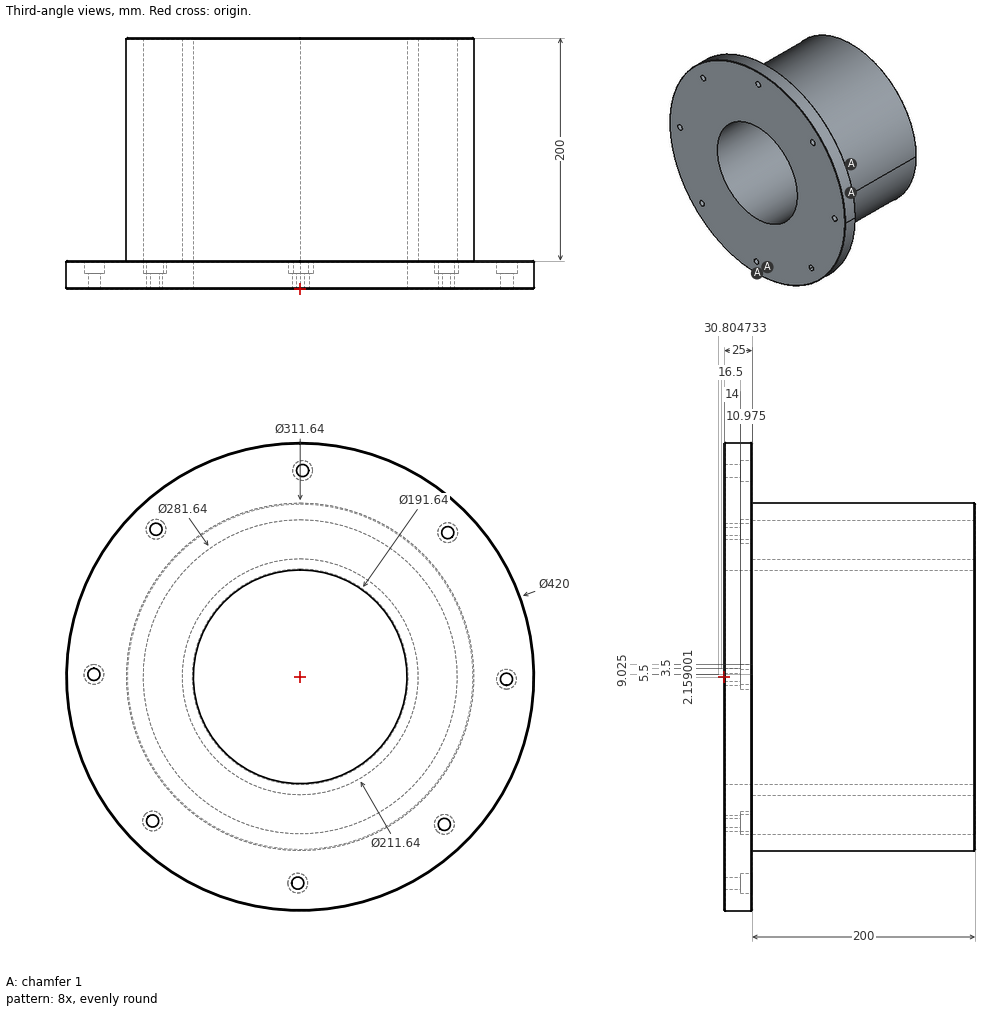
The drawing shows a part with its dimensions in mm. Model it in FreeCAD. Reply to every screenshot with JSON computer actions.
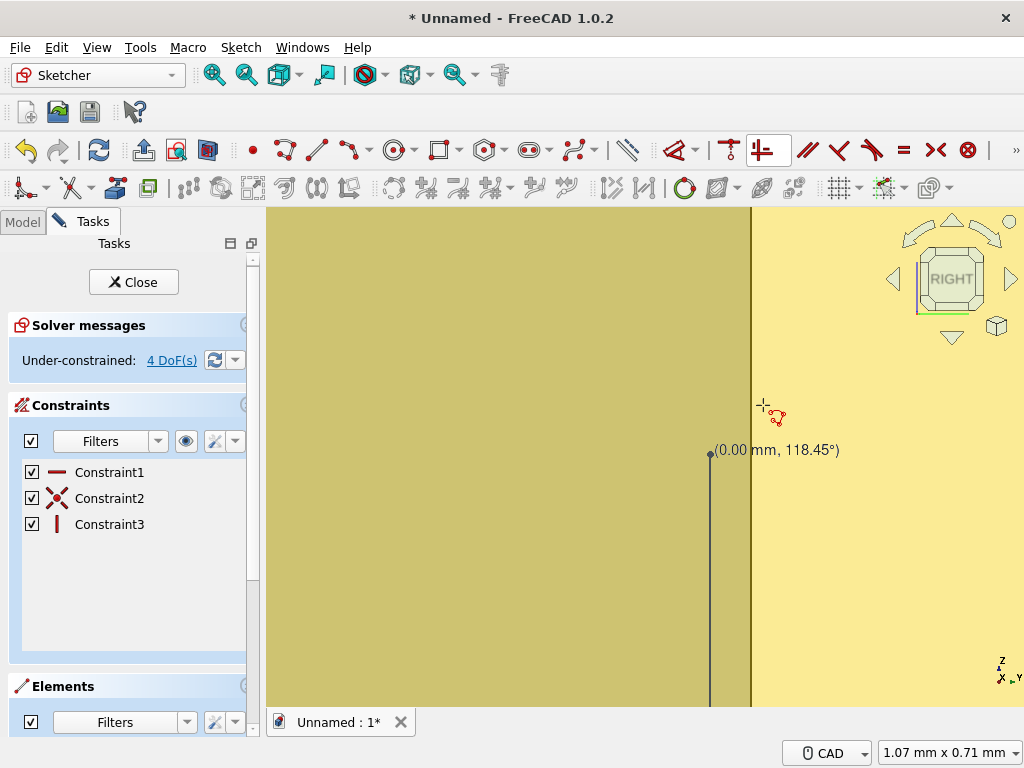
{"action": "left_click", "coordinate": [733, 398]}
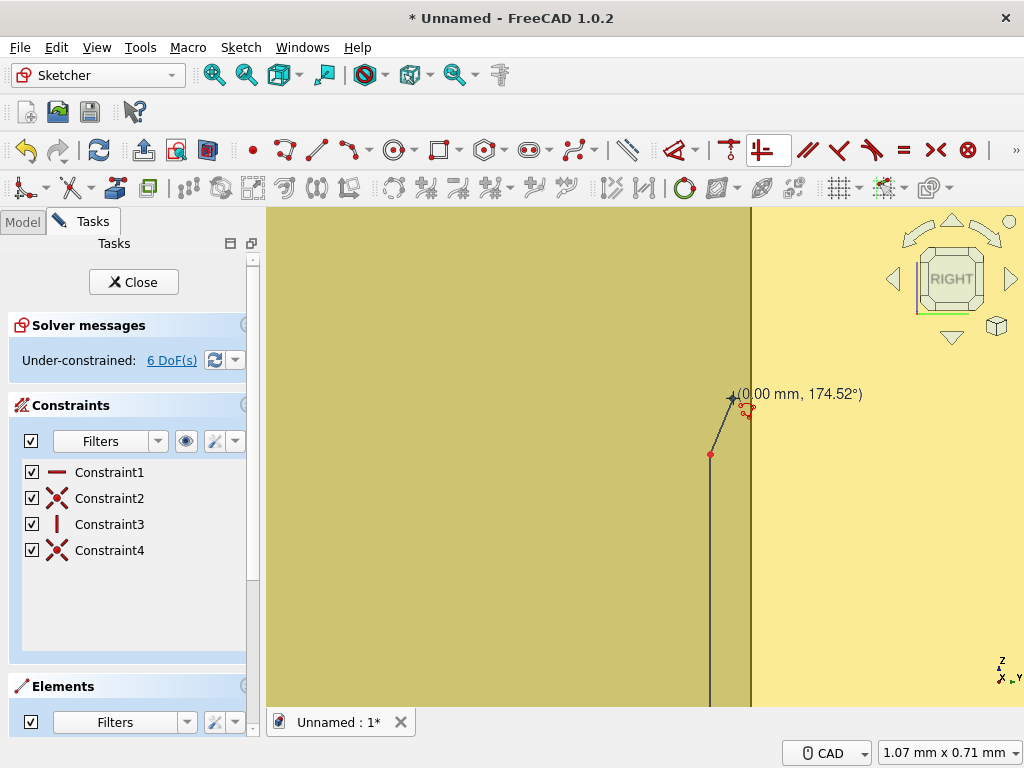
{"action": "scroll", "coordinate": [576, 457], "scroll_direction": "down", "scroll_amount": 15}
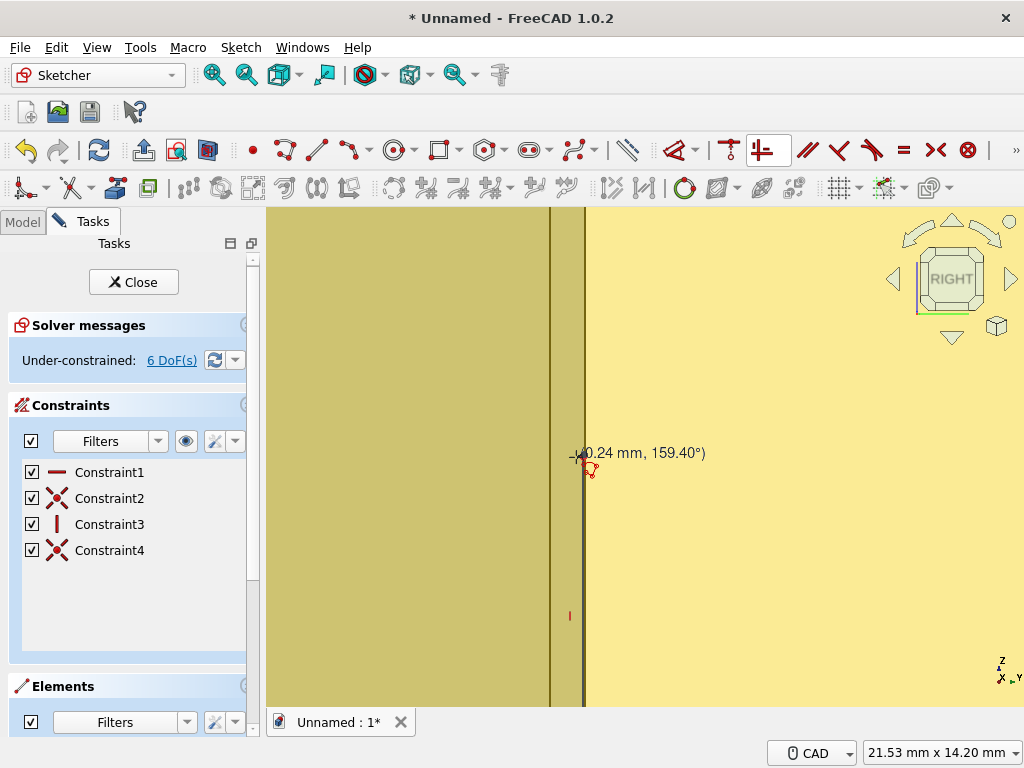
{"action": "scroll", "coordinate": [822, 394], "scroll_direction": "down", "scroll_amount": 7}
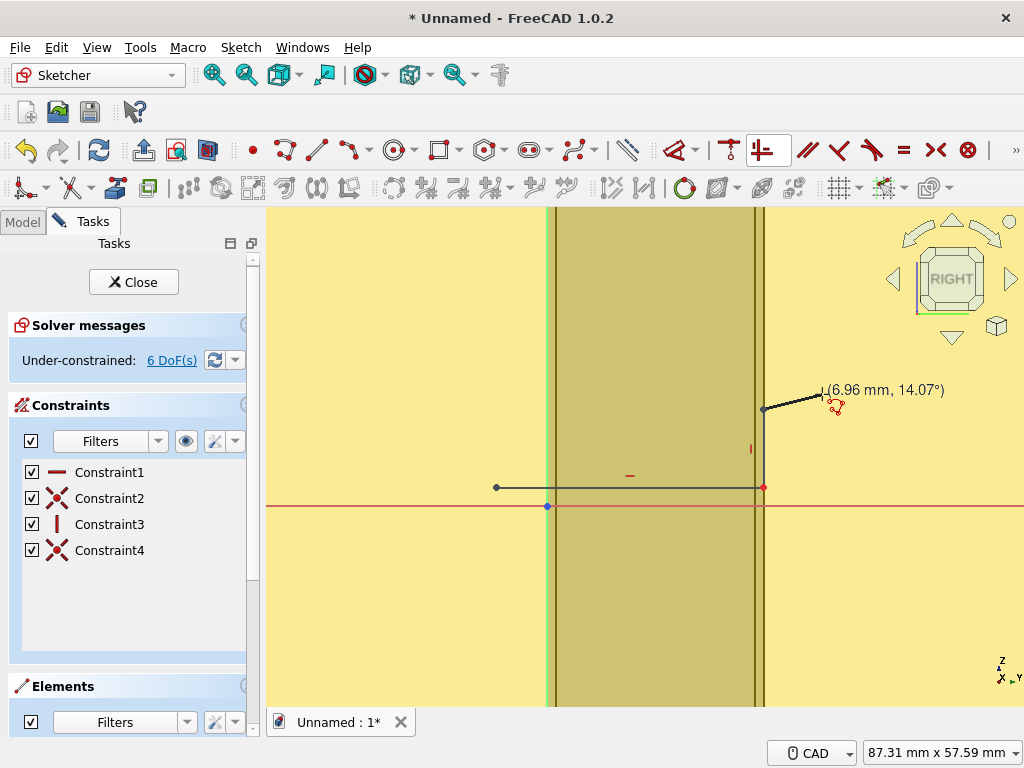
{"action": "left_click", "coordinate": [669, 409]}
{"action": "left_click", "coordinate": [669, 440]}
{"action": "left_click", "coordinate": [525, 440]}
{"action": "left_click", "coordinate": [497, 488]}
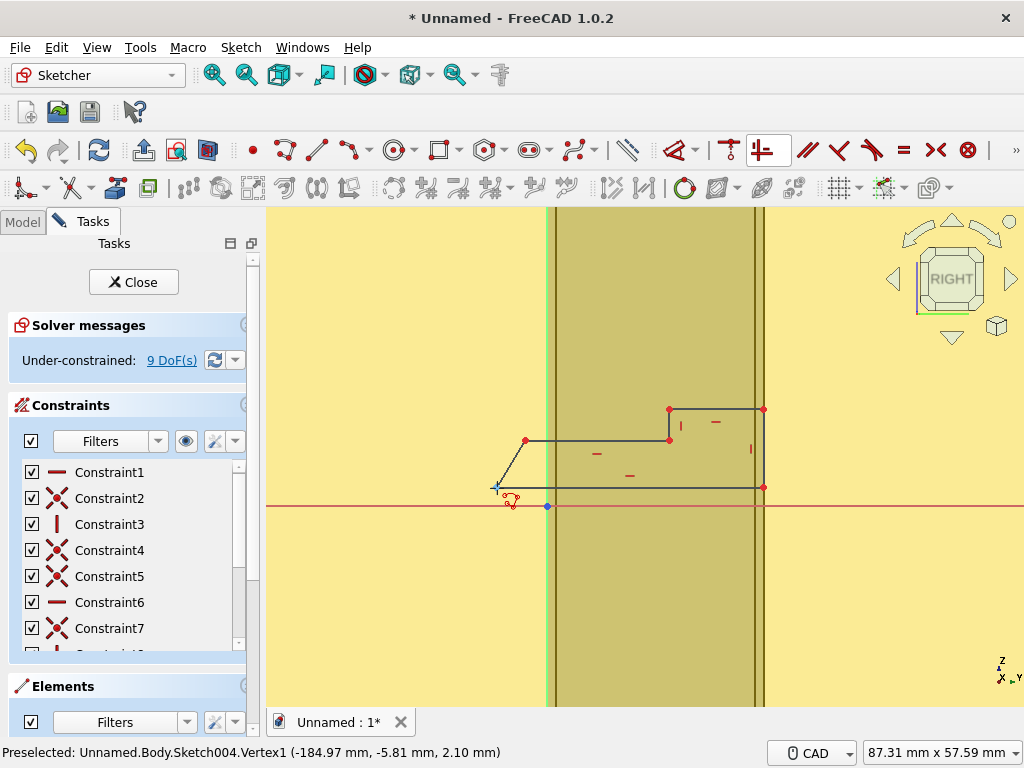
{"action": "left_click", "coordinate": [318, 150]}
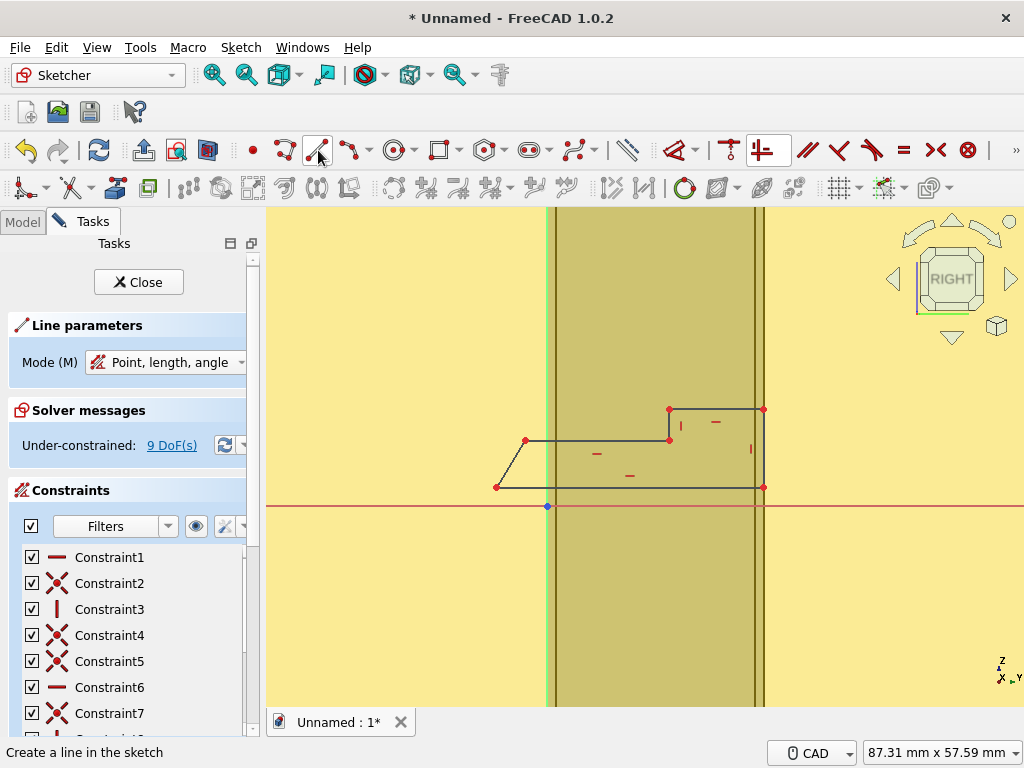
{"action": "left_click", "coordinate": [470, 487]}
{"action": "left_click", "coordinate": [390, 487]}
{"action": "key", "text": "Escape"}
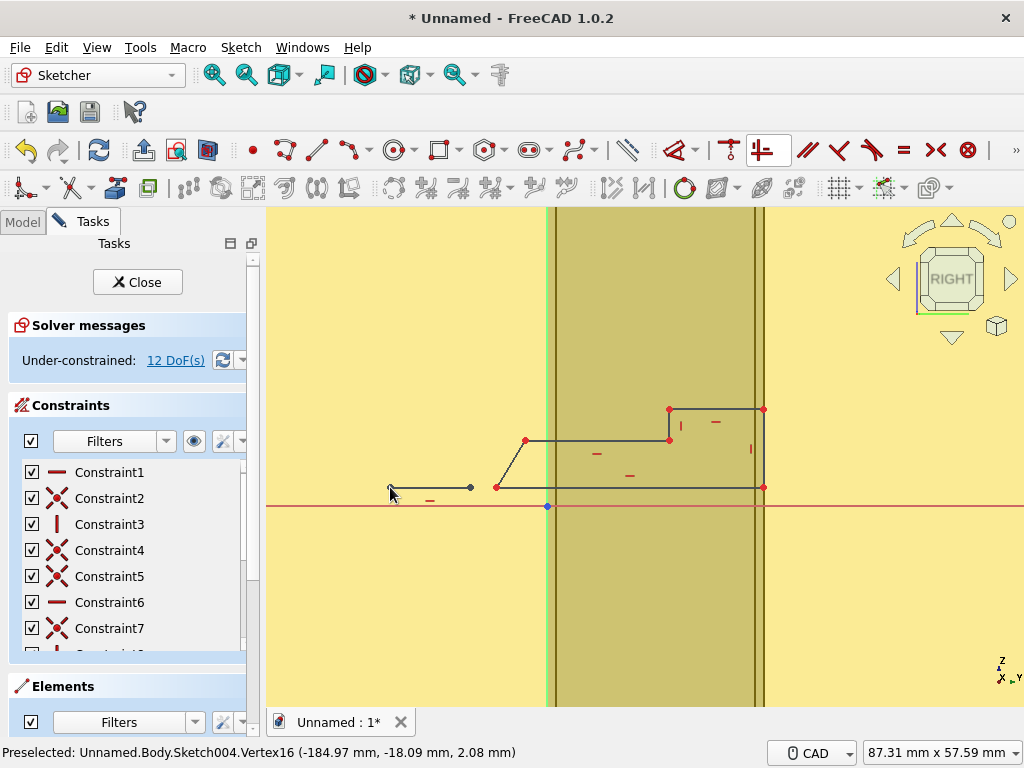
{"action": "left_click", "coordinate": [446, 488]}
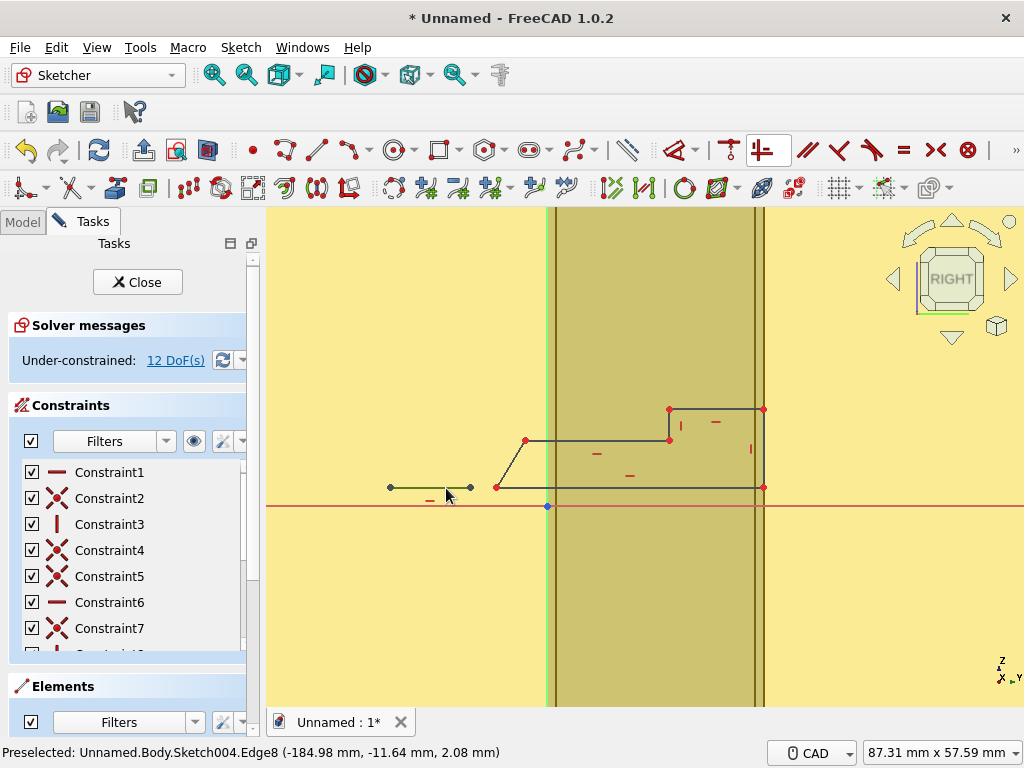
{"action": "left_click", "coordinate": [628, 150]}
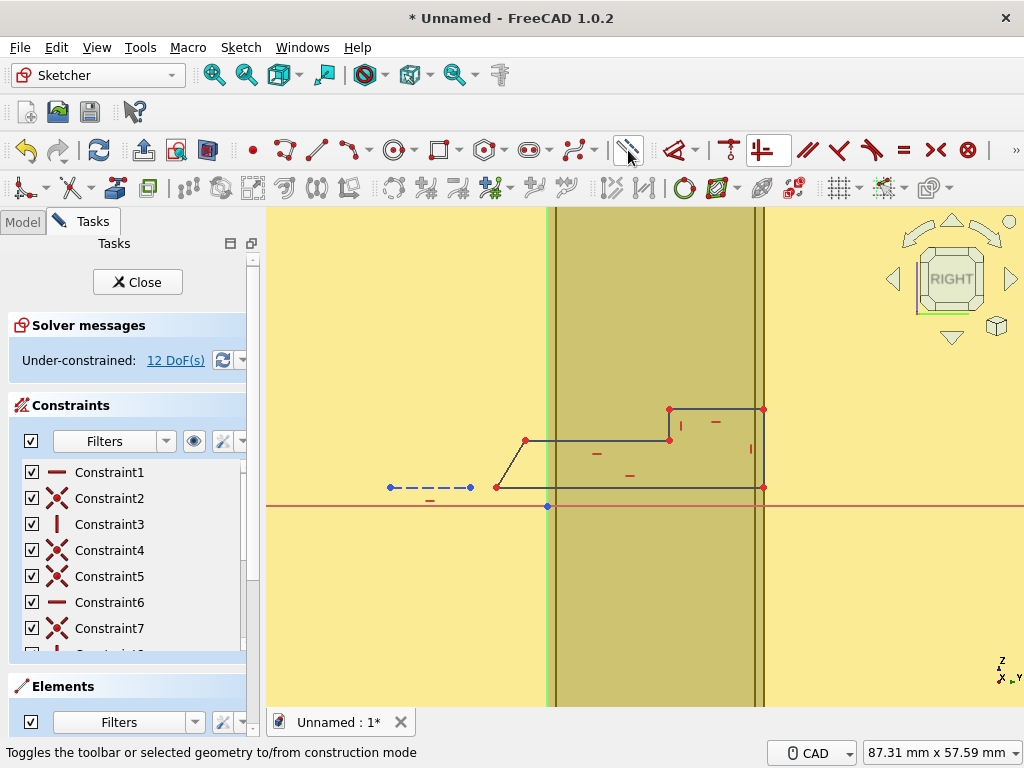
{"action": "key", "text": "d"}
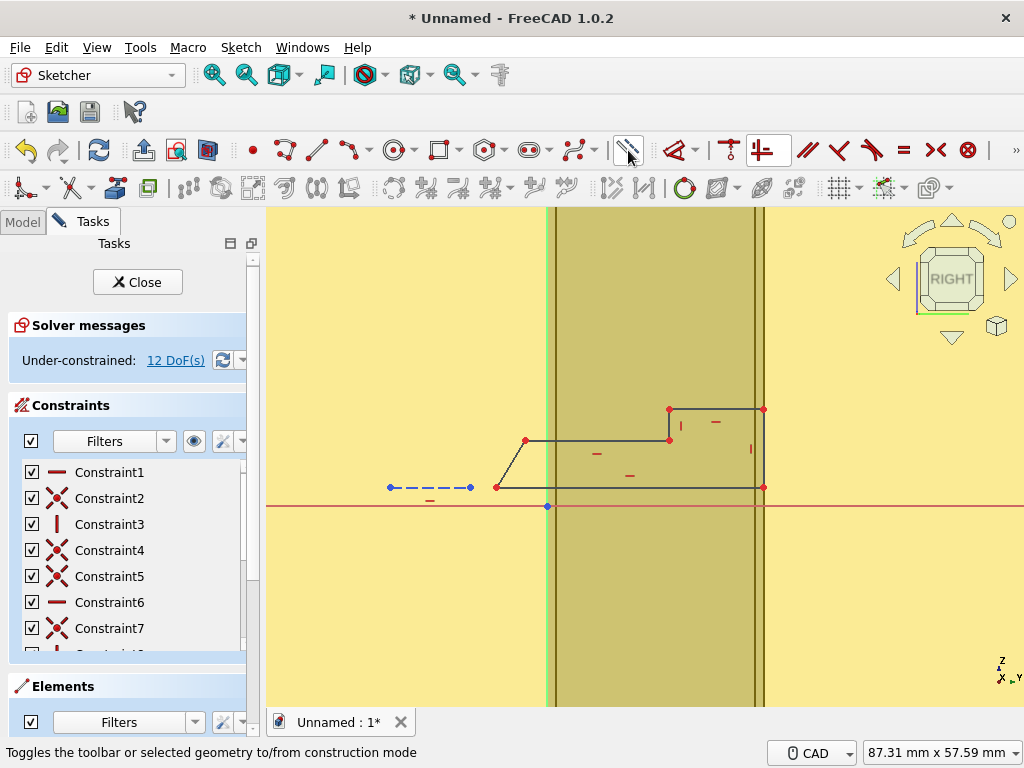
{"action": "scroll", "coordinate": [669, 419], "scroll_direction": "up", "scroll_amount": 2}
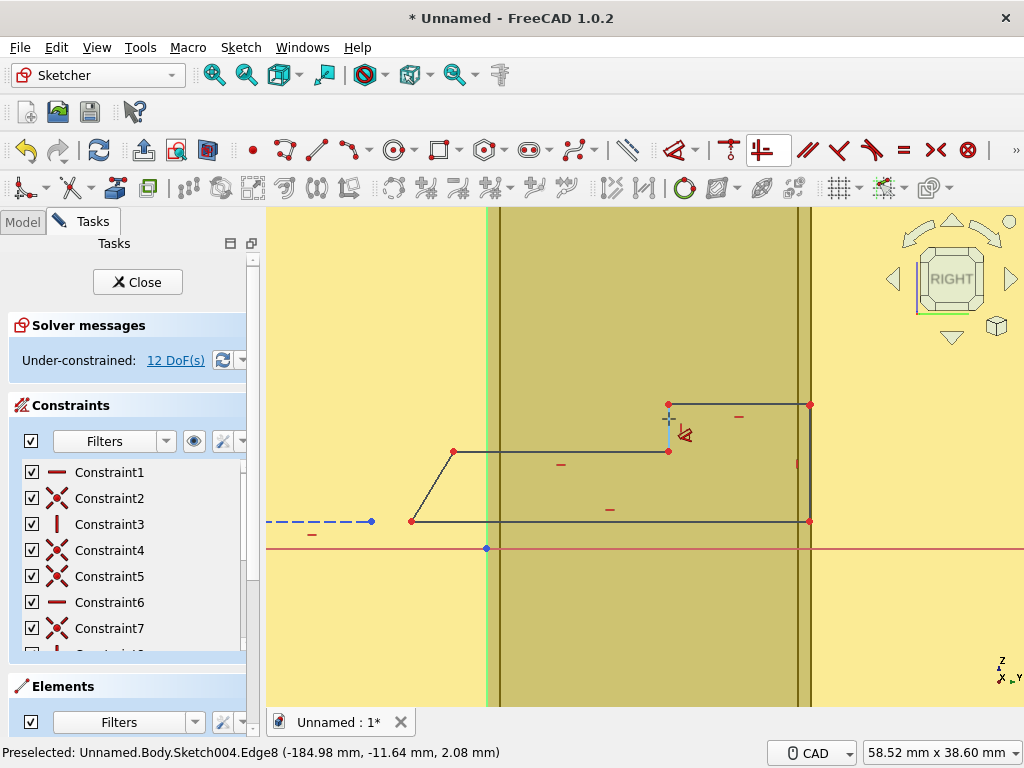
{"action": "left_click", "coordinate": [669, 418]}
{"action": "left_click", "coordinate": [703, 428]}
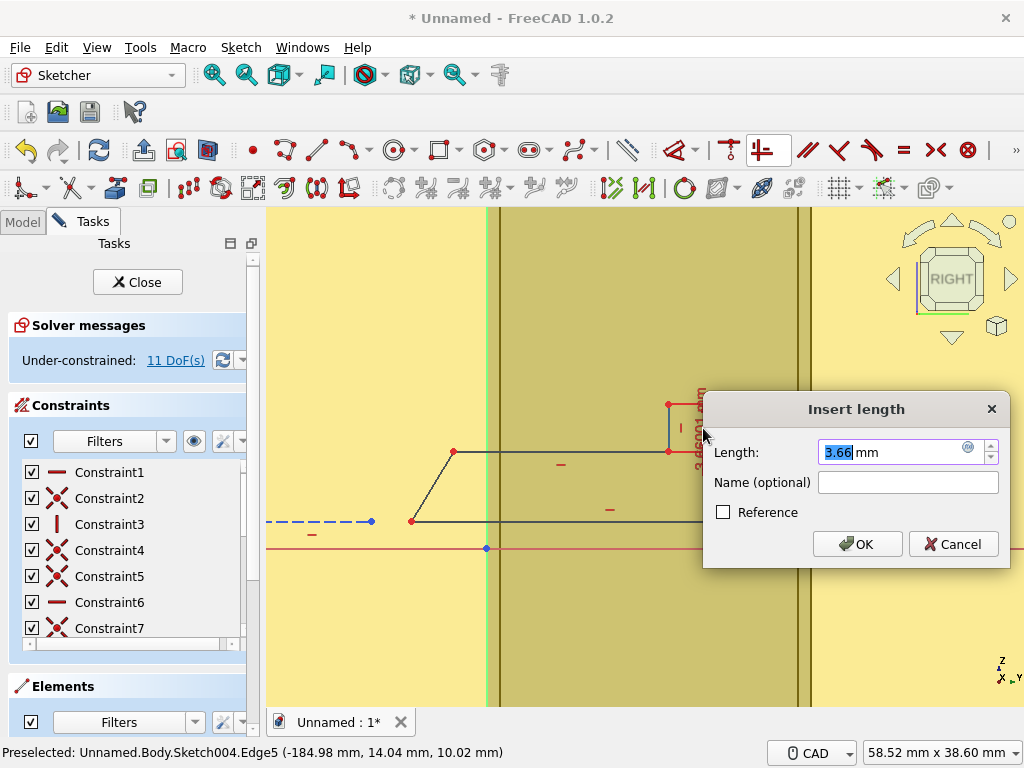
{"action": "type", "text": "3.5"}
{"action": "key", "text": "Return"}